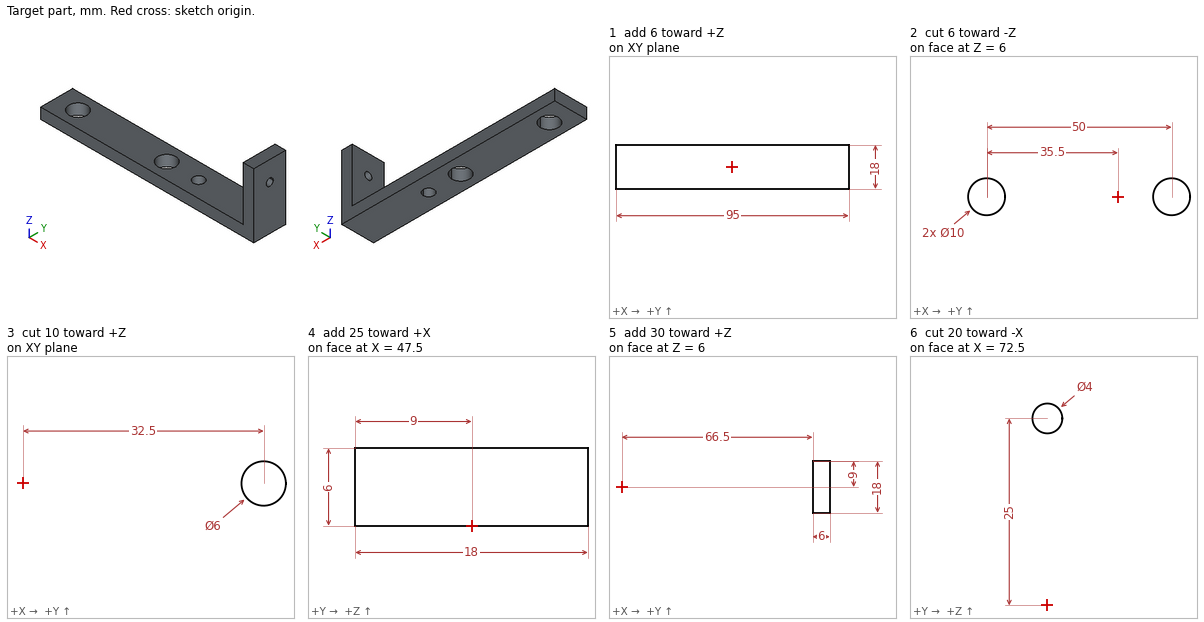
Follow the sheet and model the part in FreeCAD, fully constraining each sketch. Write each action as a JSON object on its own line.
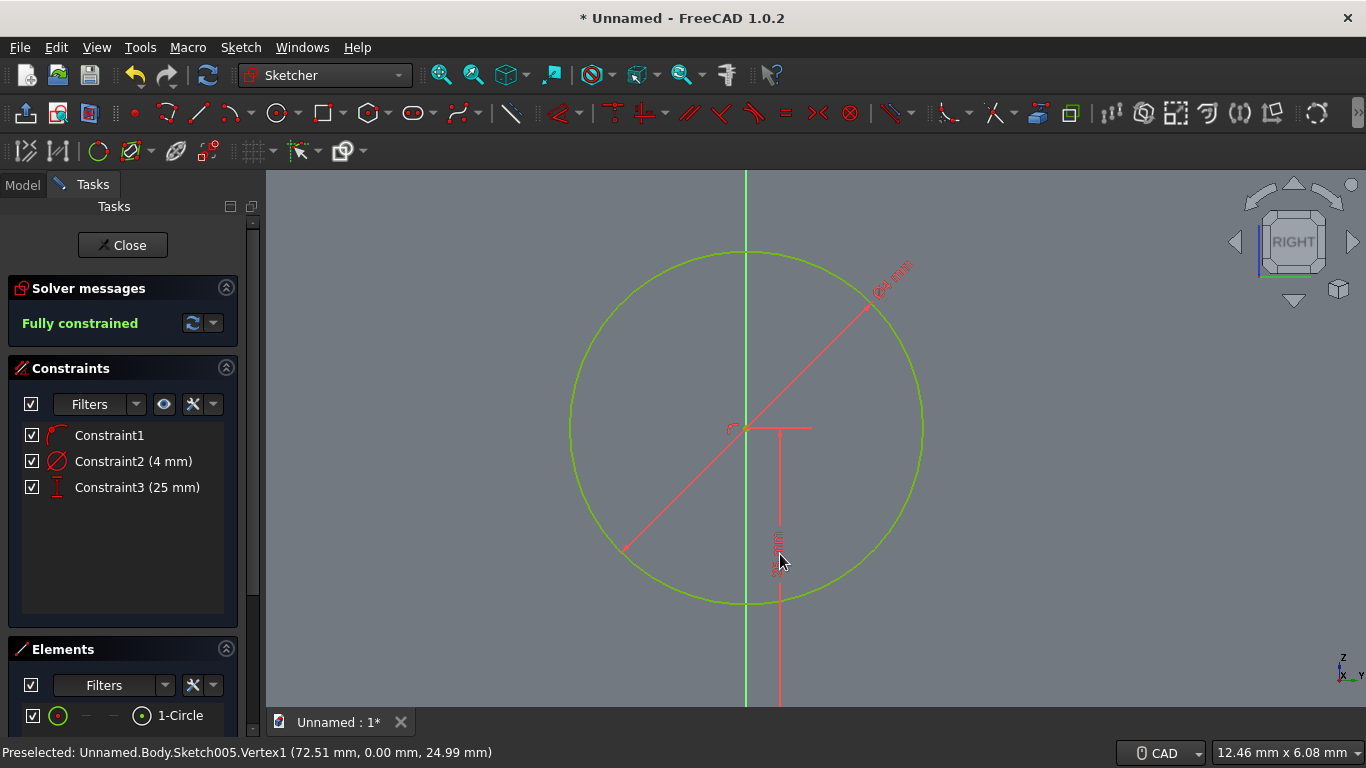
{"action": "left_click", "coordinate": [123, 245]}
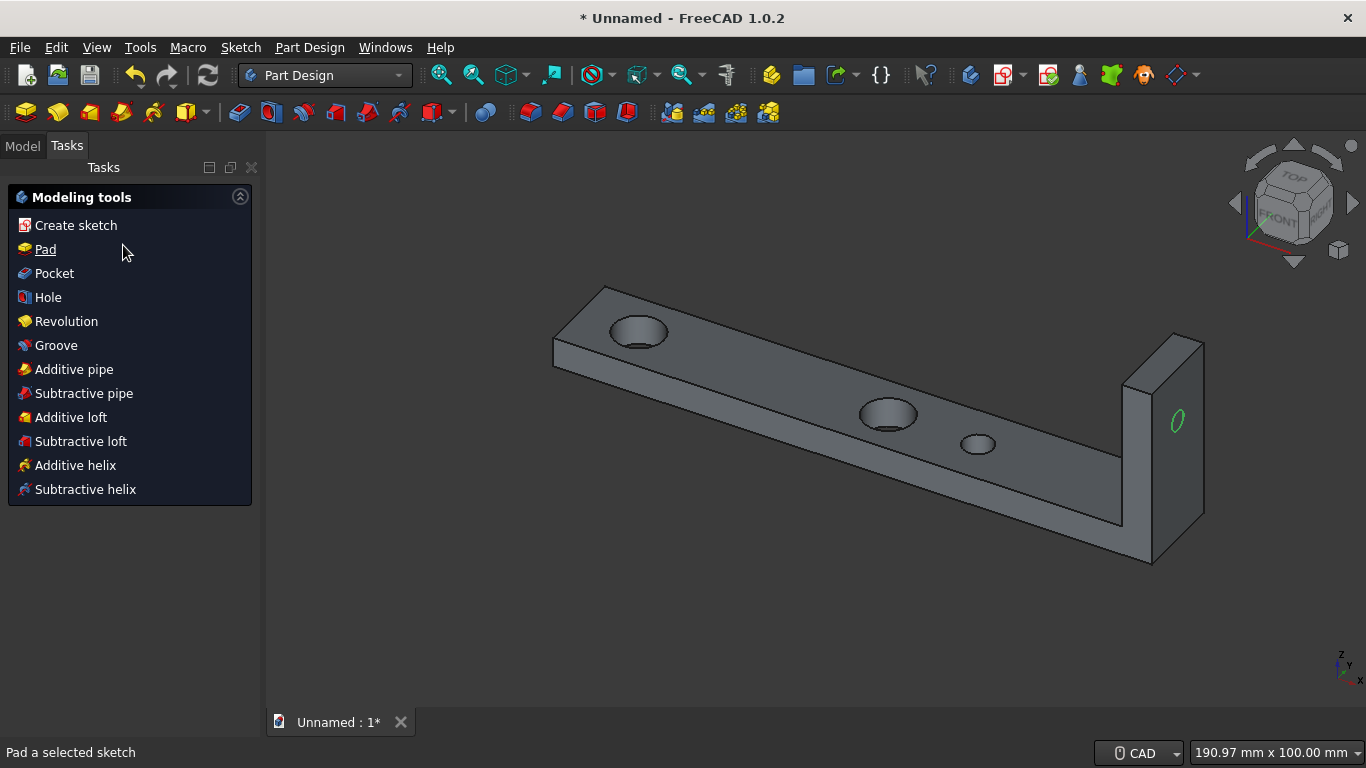
{"action": "left_click", "coordinate": [240, 112]}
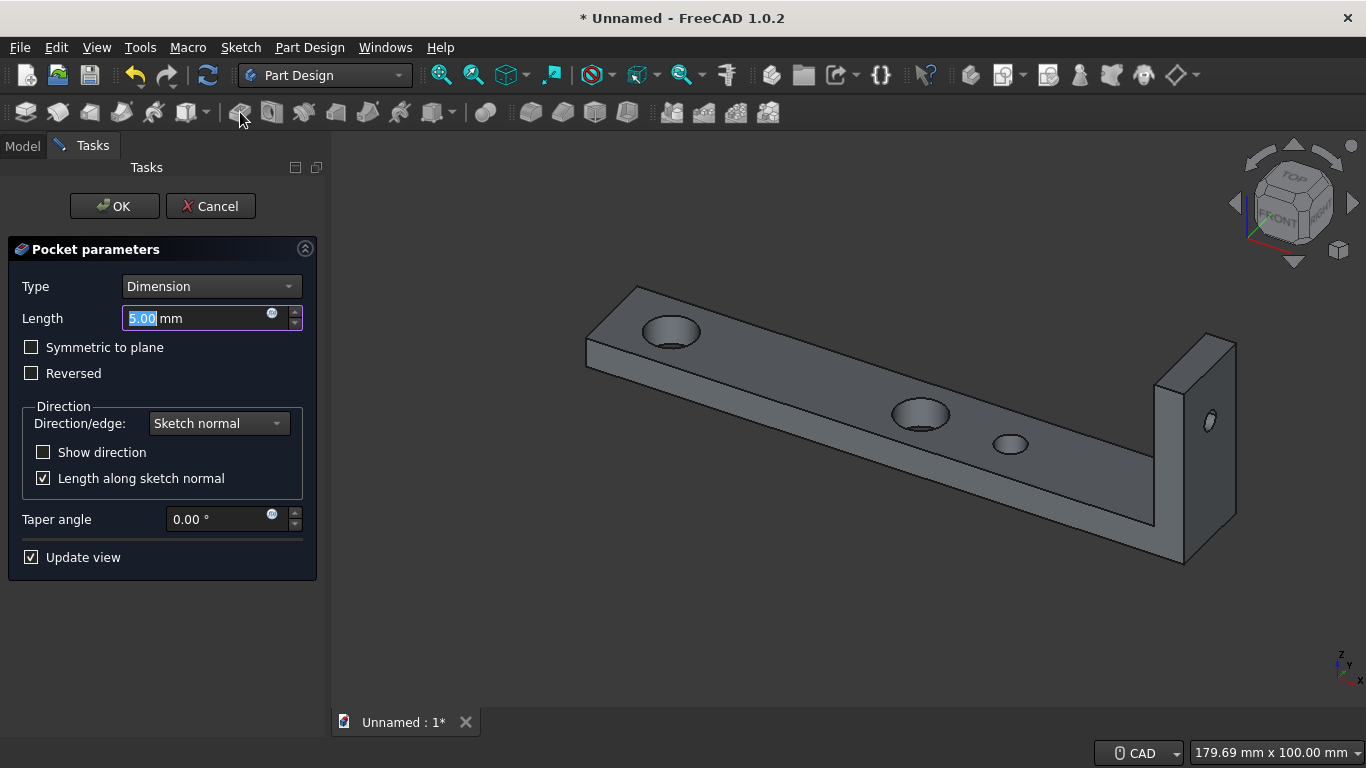
{"action": "type", "text": "20"}
{"action": "key", "text": "Tab"}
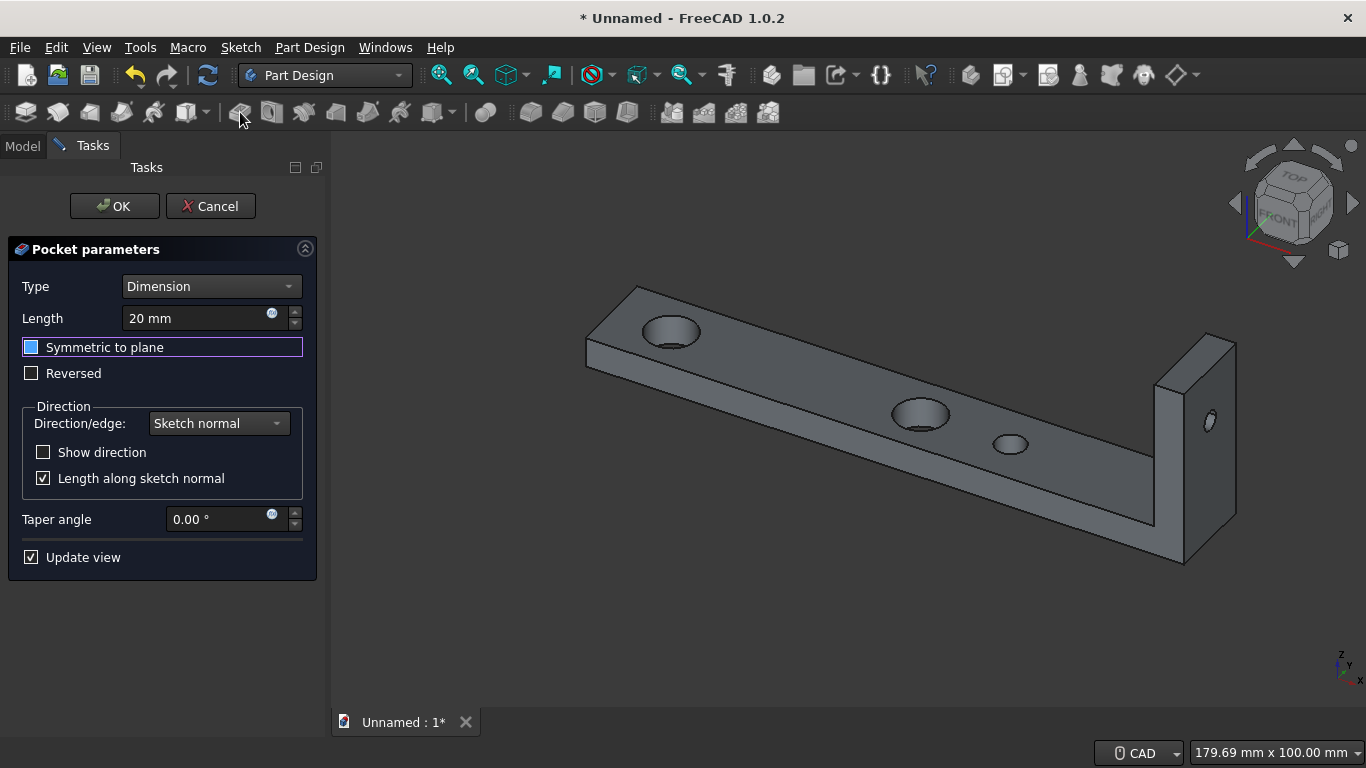
{"action": "left_click", "coordinate": [115, 206]}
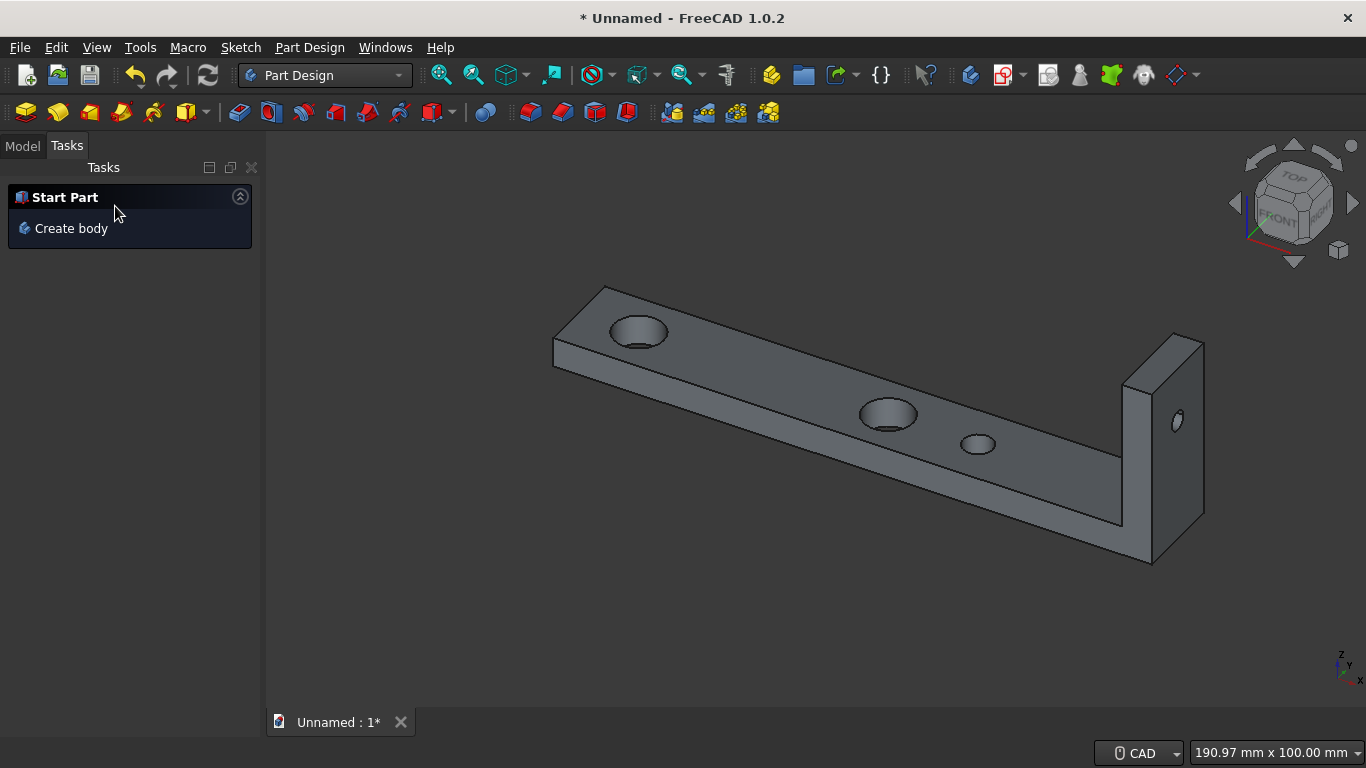
{"action": "key", "text": "0"}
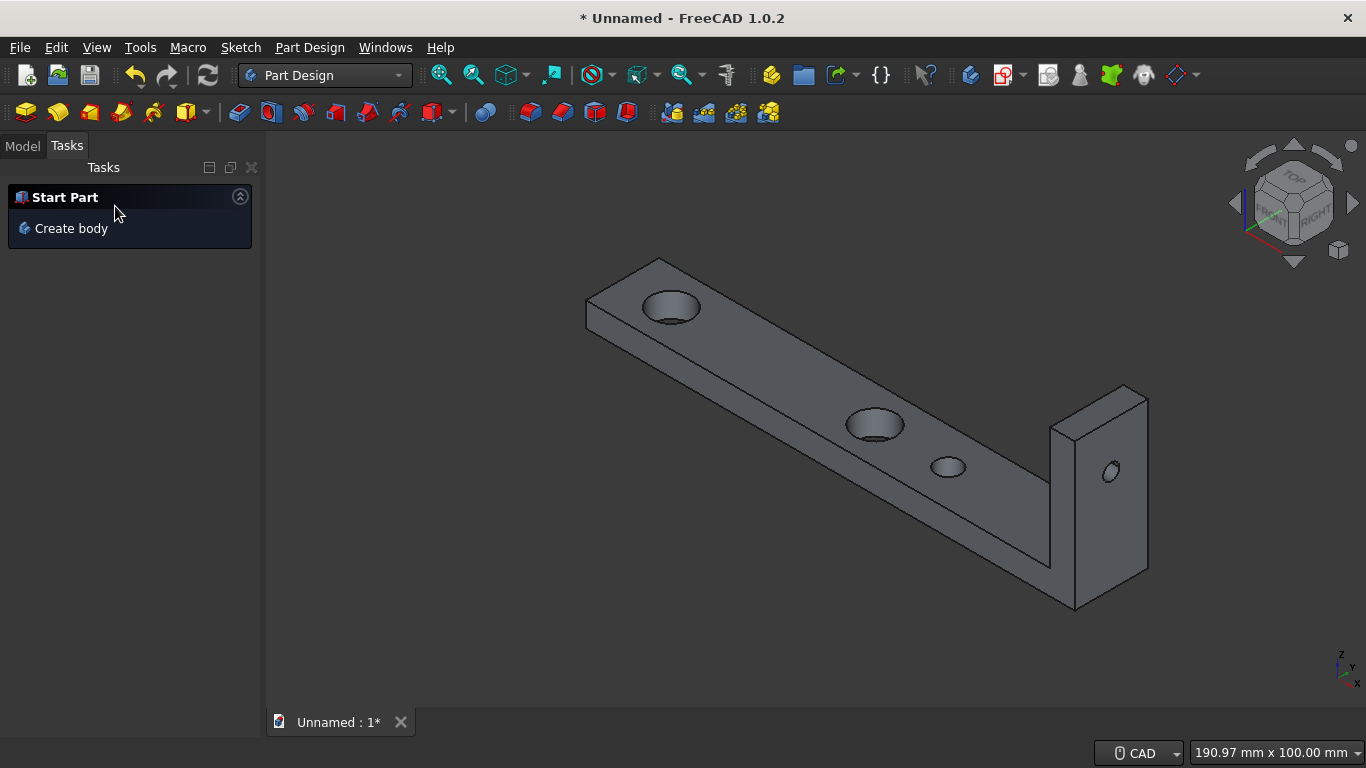
{"action": "left_click", "coordinate": [442, 76]}